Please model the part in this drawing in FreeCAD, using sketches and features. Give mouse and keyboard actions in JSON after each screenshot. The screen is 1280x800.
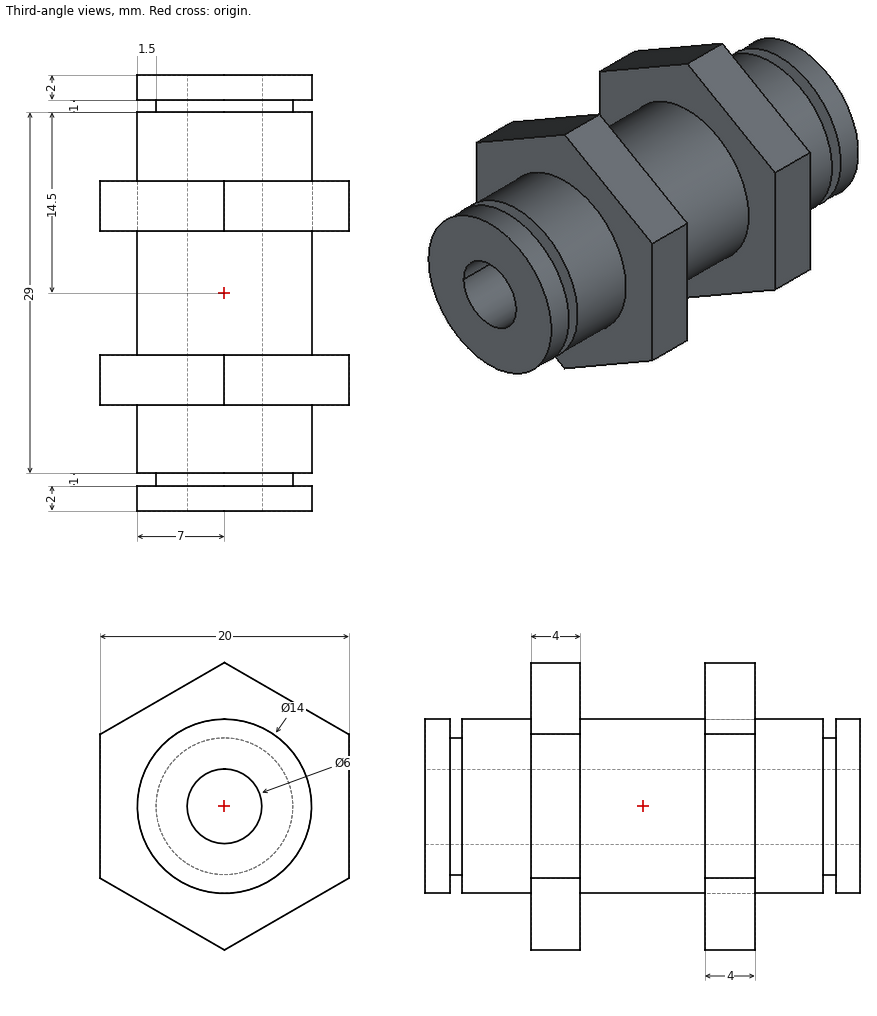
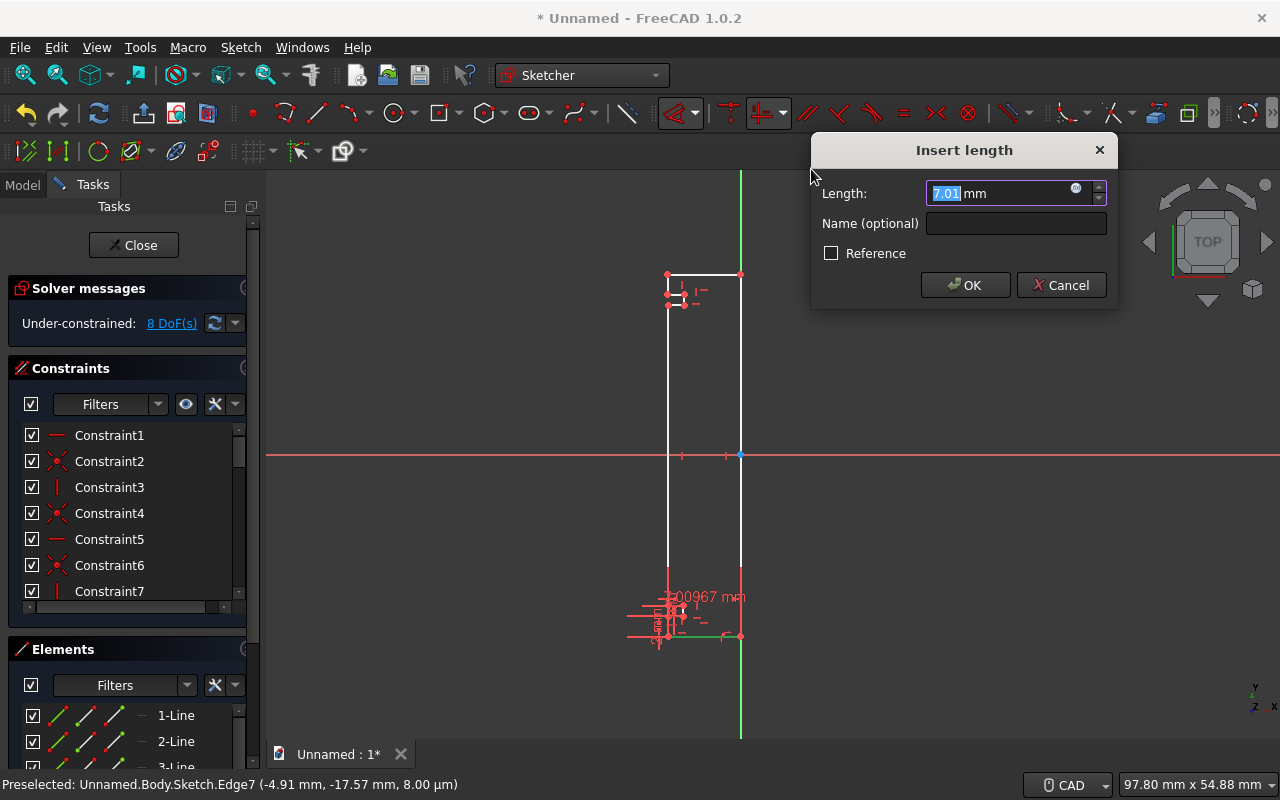
{"action": "type", "text": "7"}
{"action": "key", "text": "Return"}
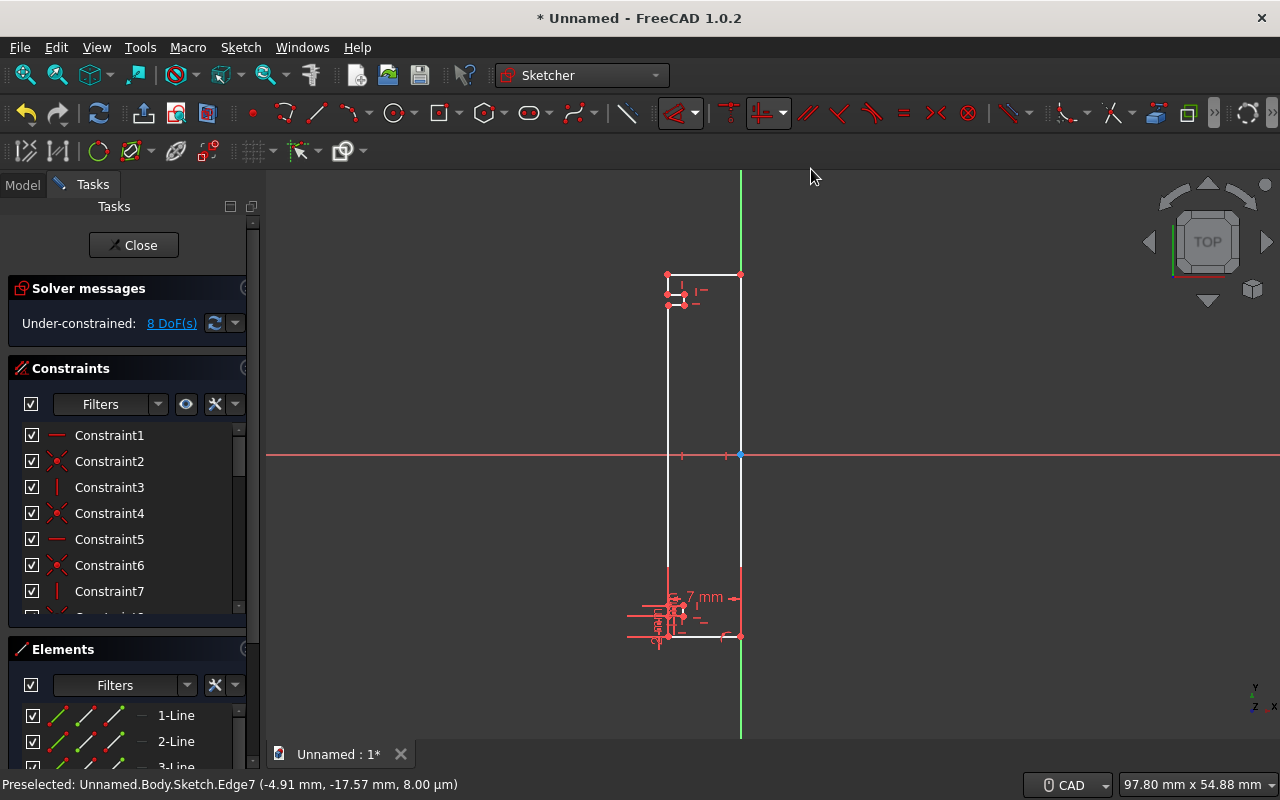
{"action": "left_click", "coordinate": [719, 275]}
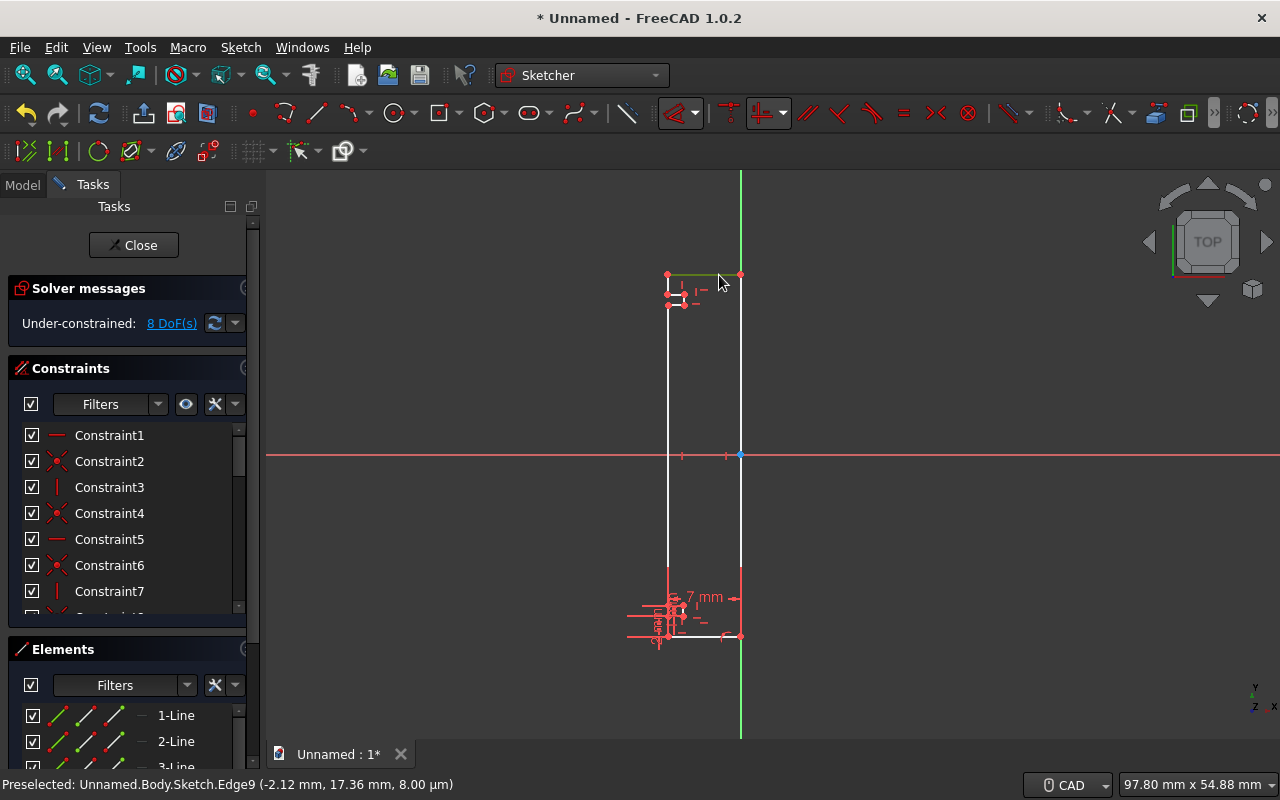
{"action": "key", "text": "l"}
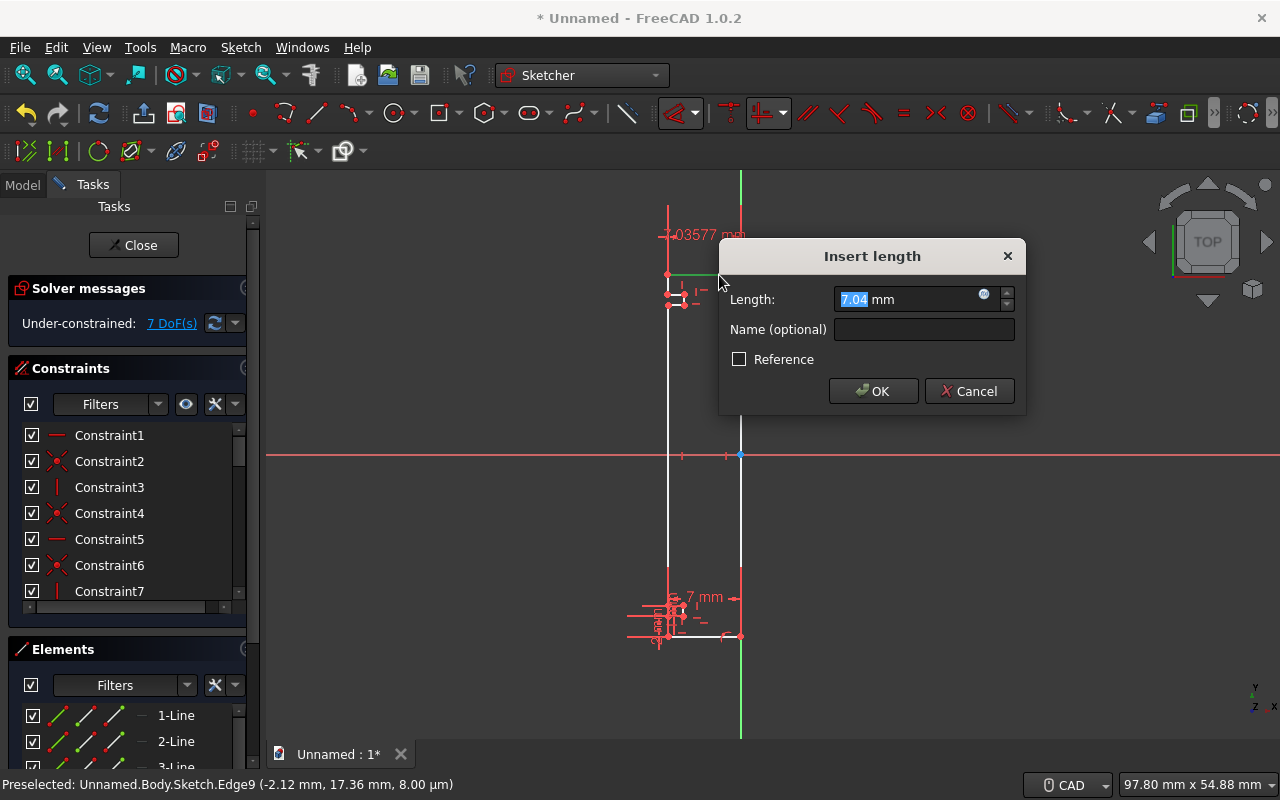
{"action": "type", "text": "7"}
{"action": "key", "text": "Return"}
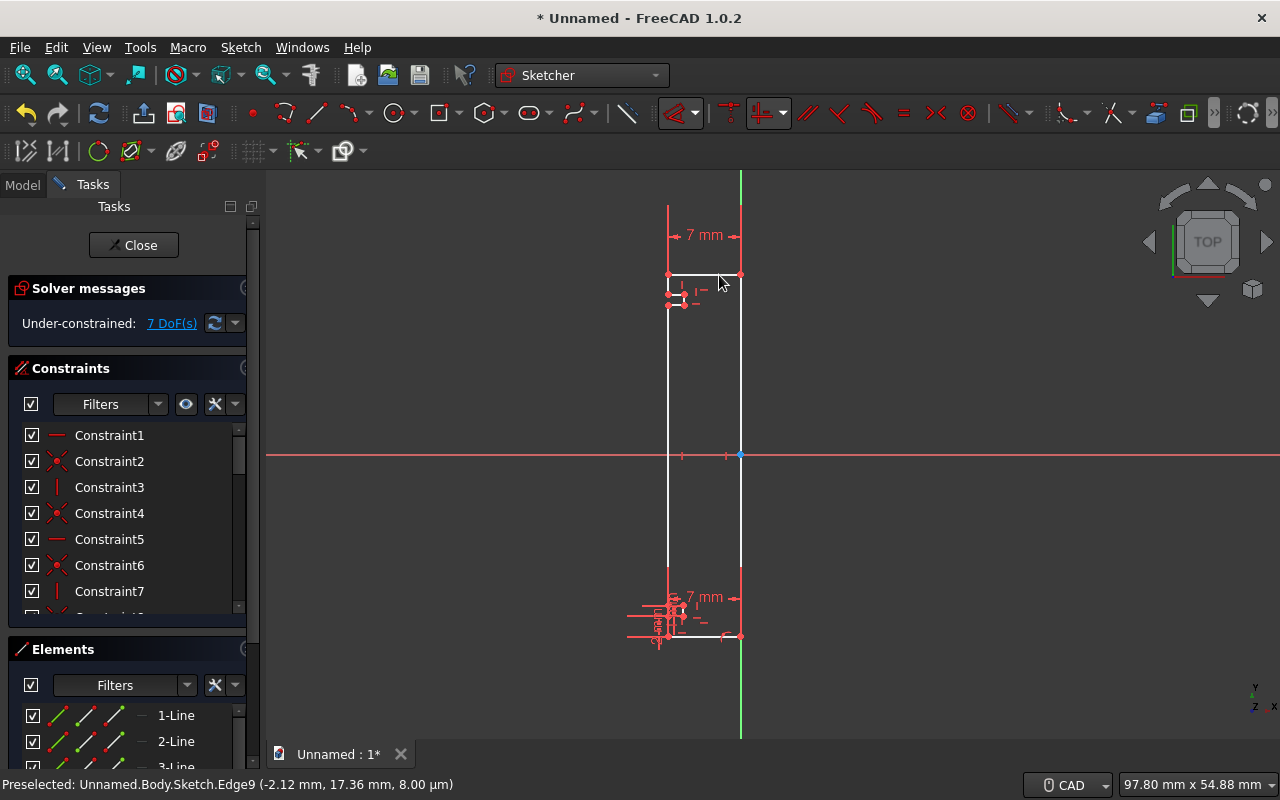
{"action": "scroll", "coordinate": [668, 285], "scroll_direction": "up", "scroll_amount": 4}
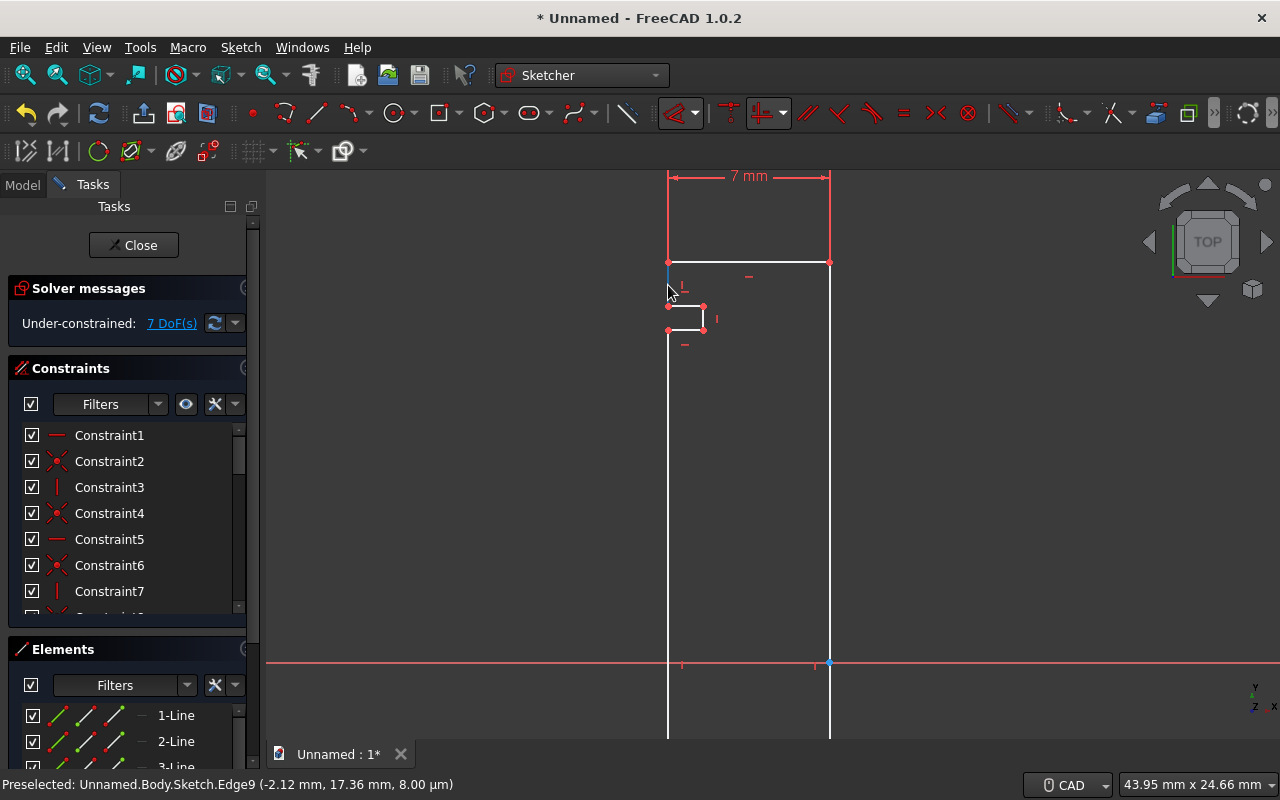
{"action": "left_click", "coordinate": [668, 284]}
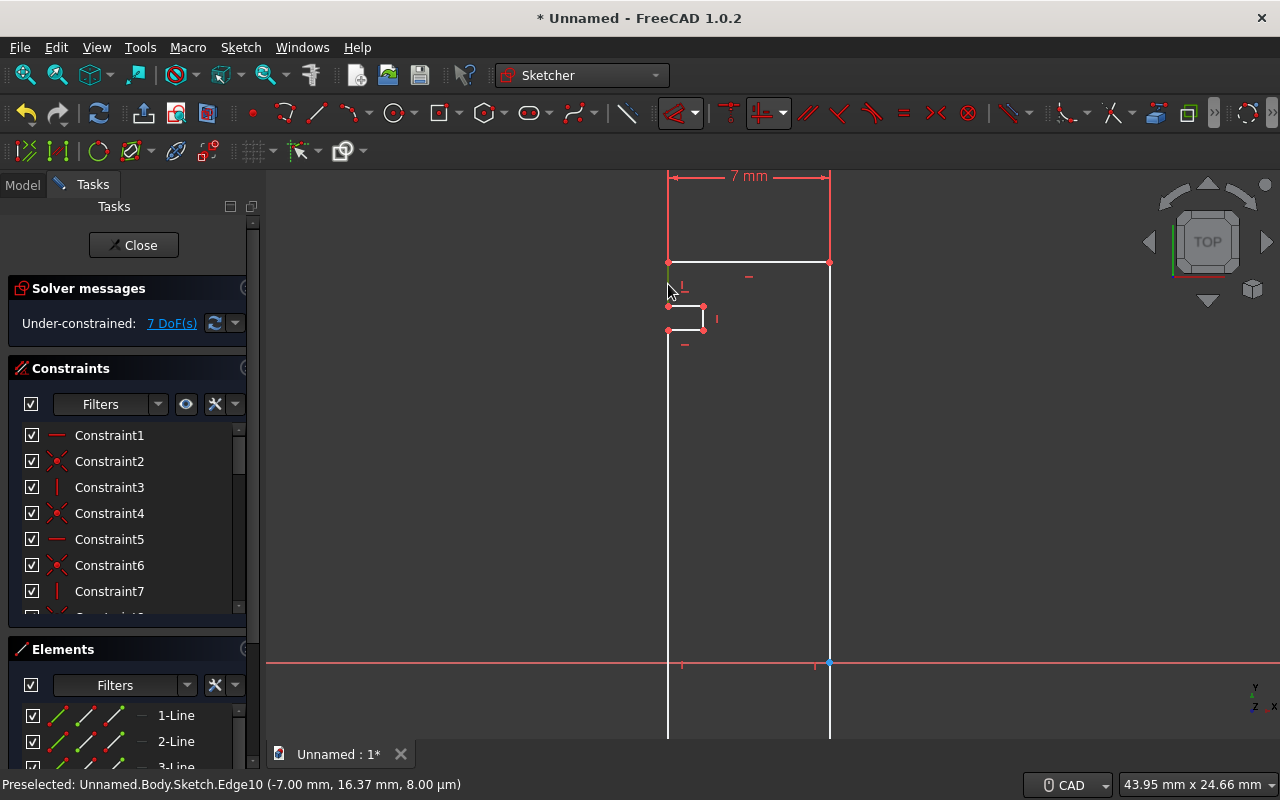
{"action": "left_click", "coordinate": [698, 114]}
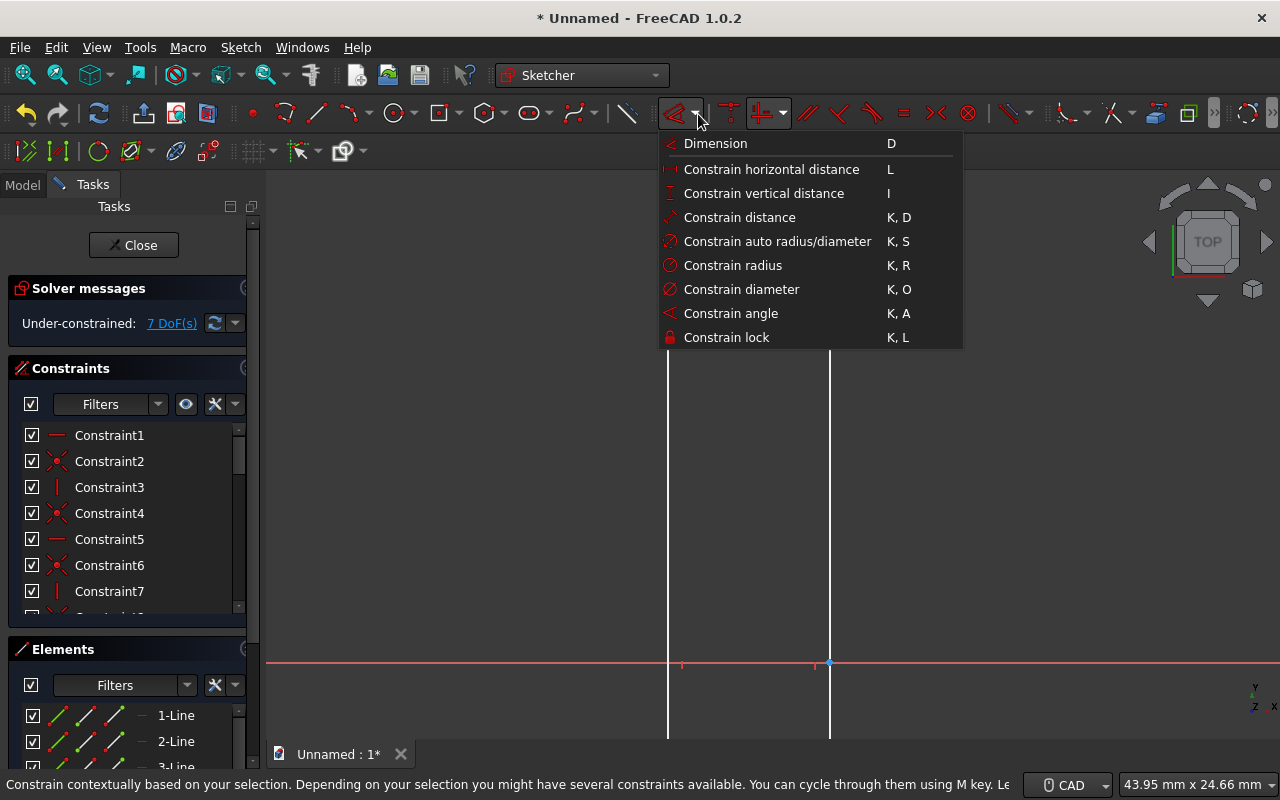
{"action": "left_click", "coordinate": [811, 193]}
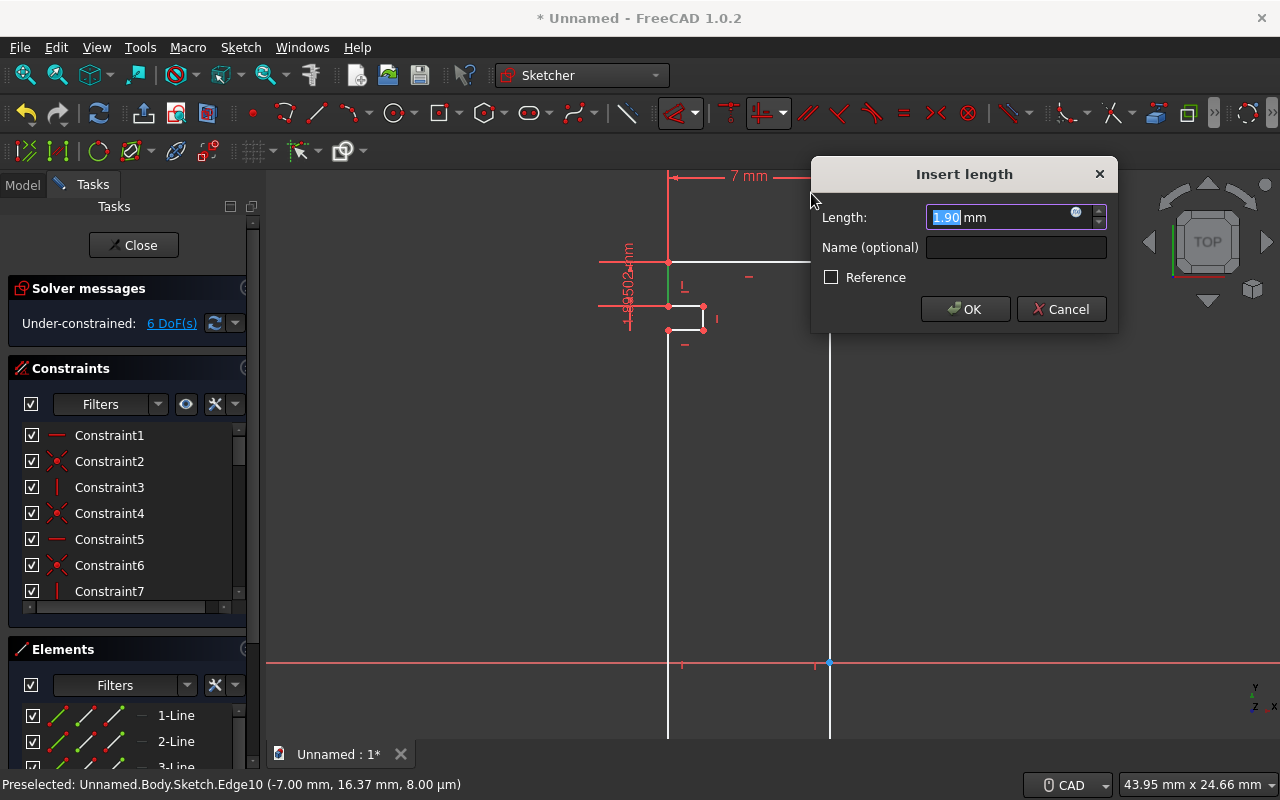
{"action": "type", "text": "2"}
{"action": "key", "text": "Return"}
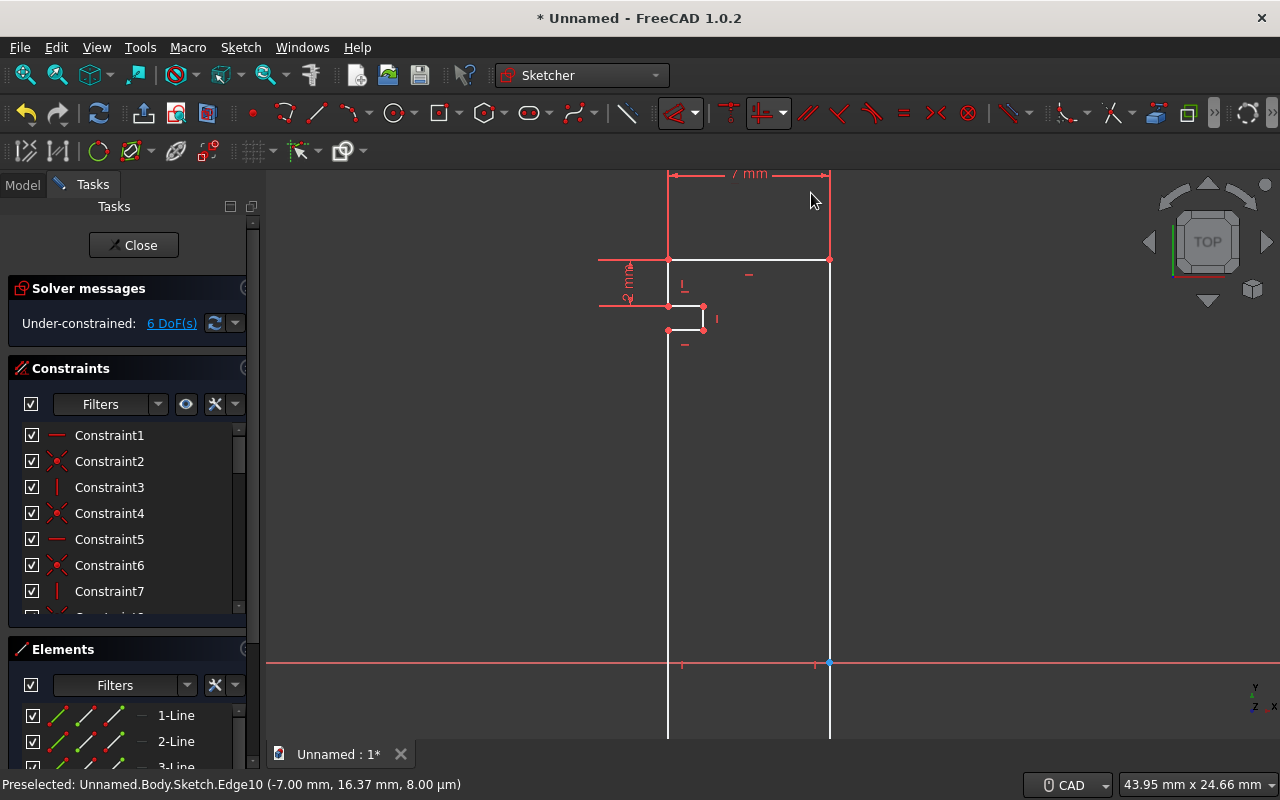
{"action": "scroll", "coordinate": [703, 316], "scroll_direction": "up", "scroll_amount": 3}